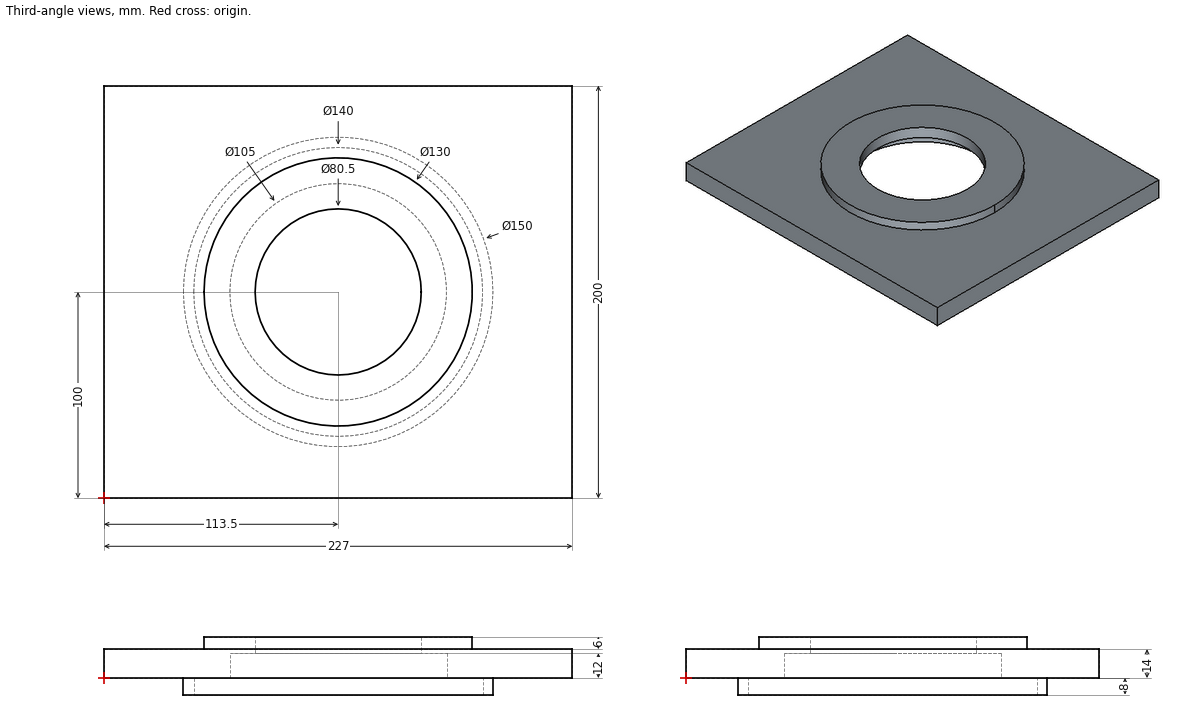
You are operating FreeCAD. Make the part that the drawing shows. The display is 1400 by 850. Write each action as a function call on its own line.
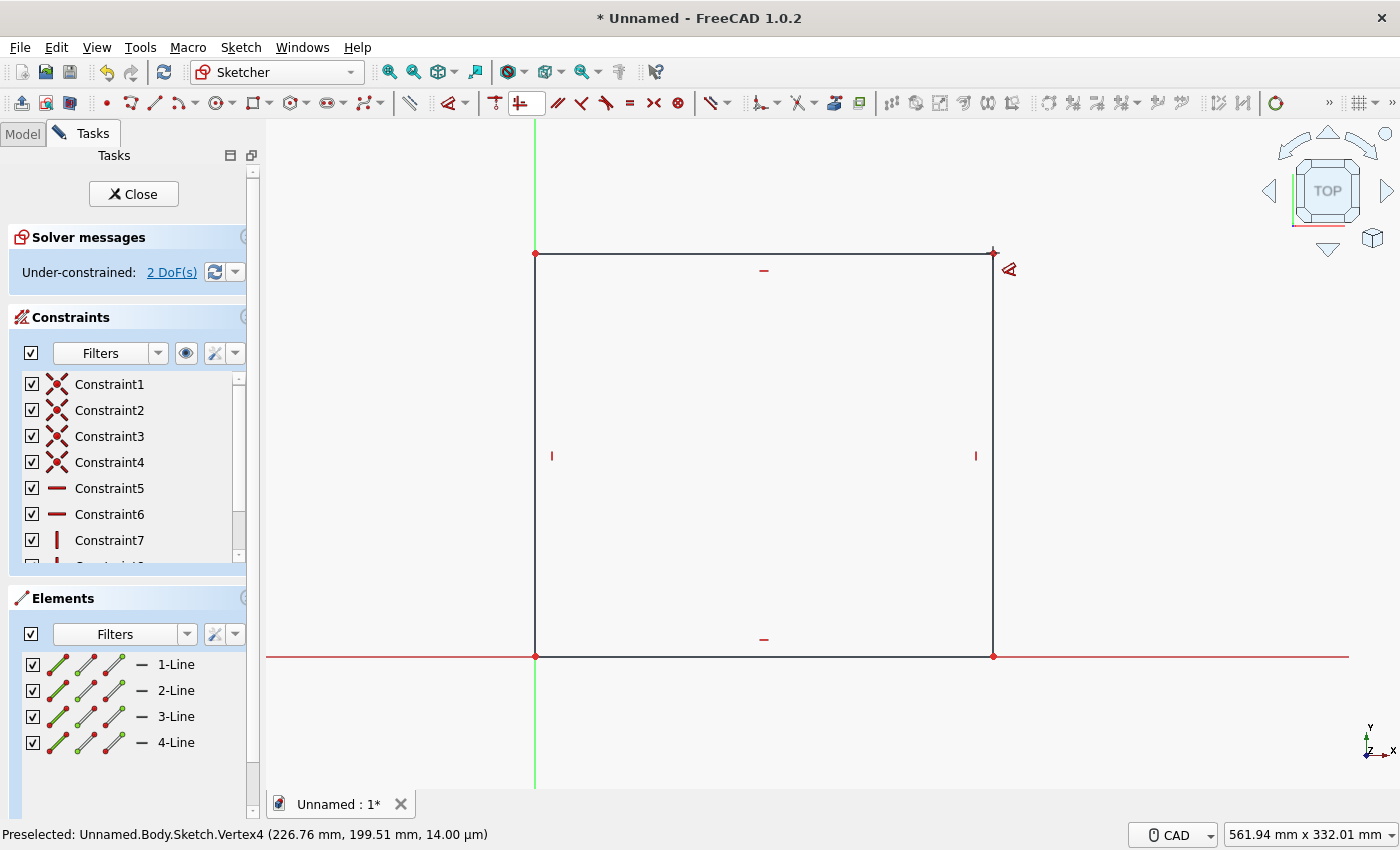
click(673, 657)
click(764, 691)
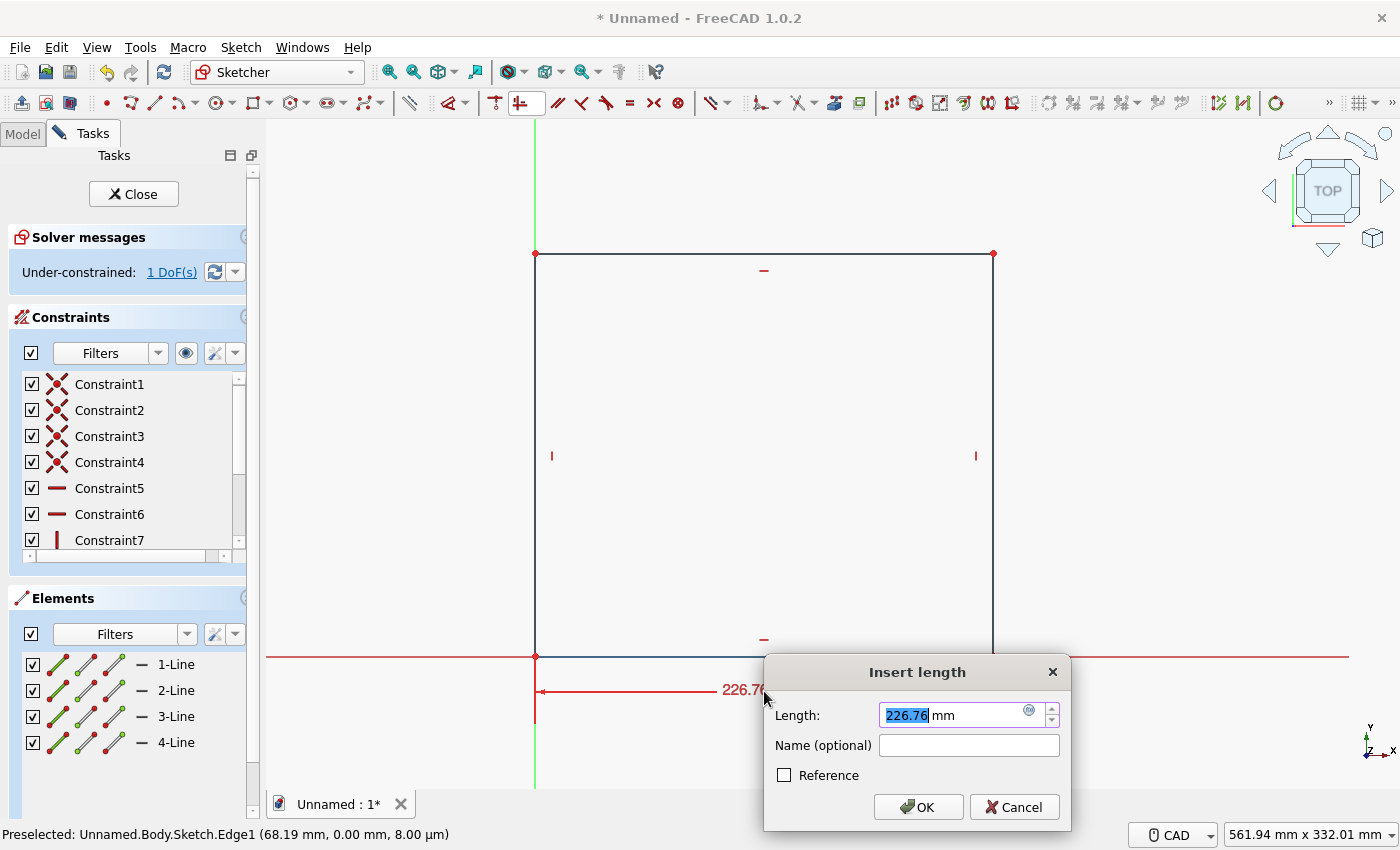
text(227)
key(Return)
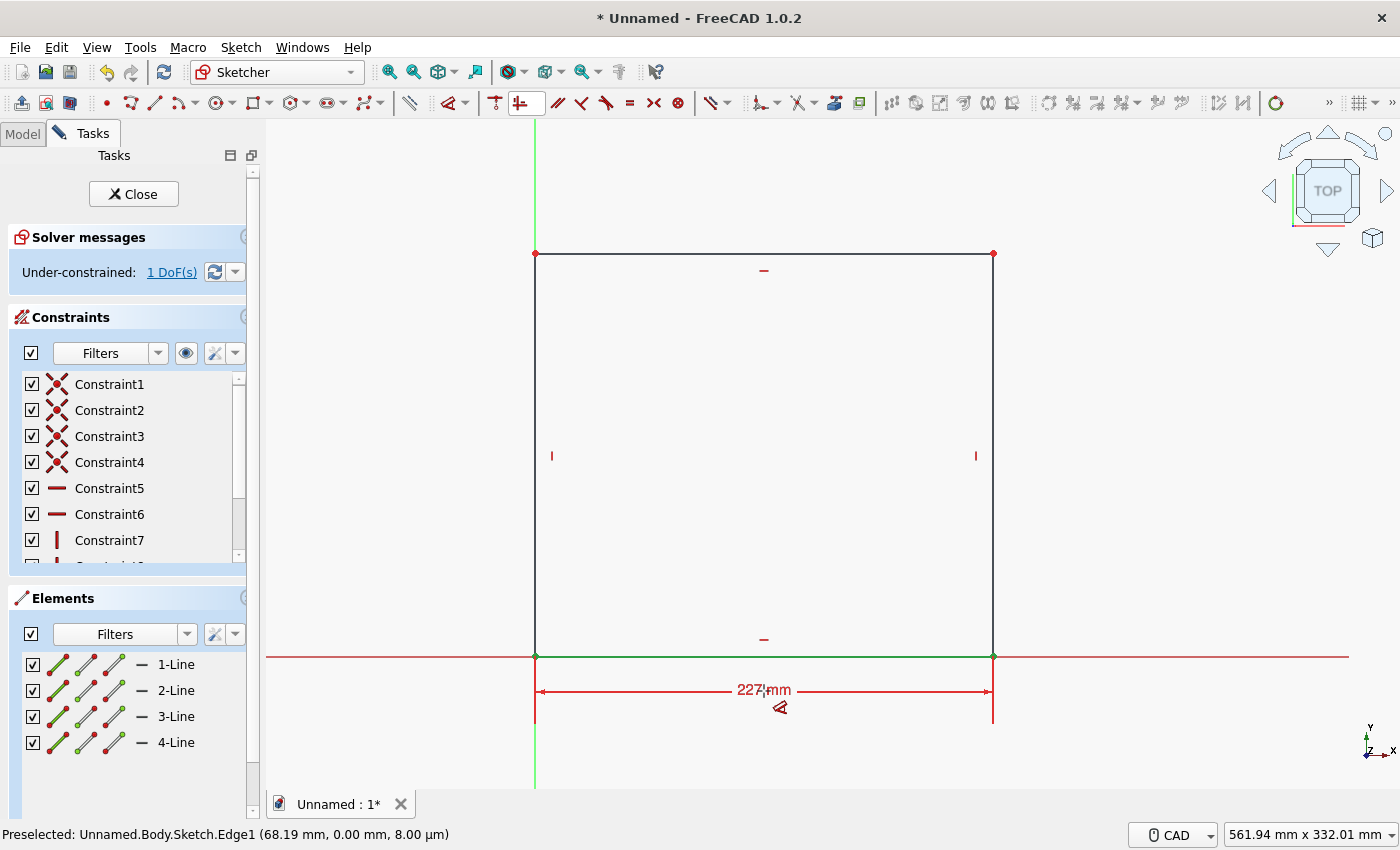
click(993, 536)
click(1027, 455)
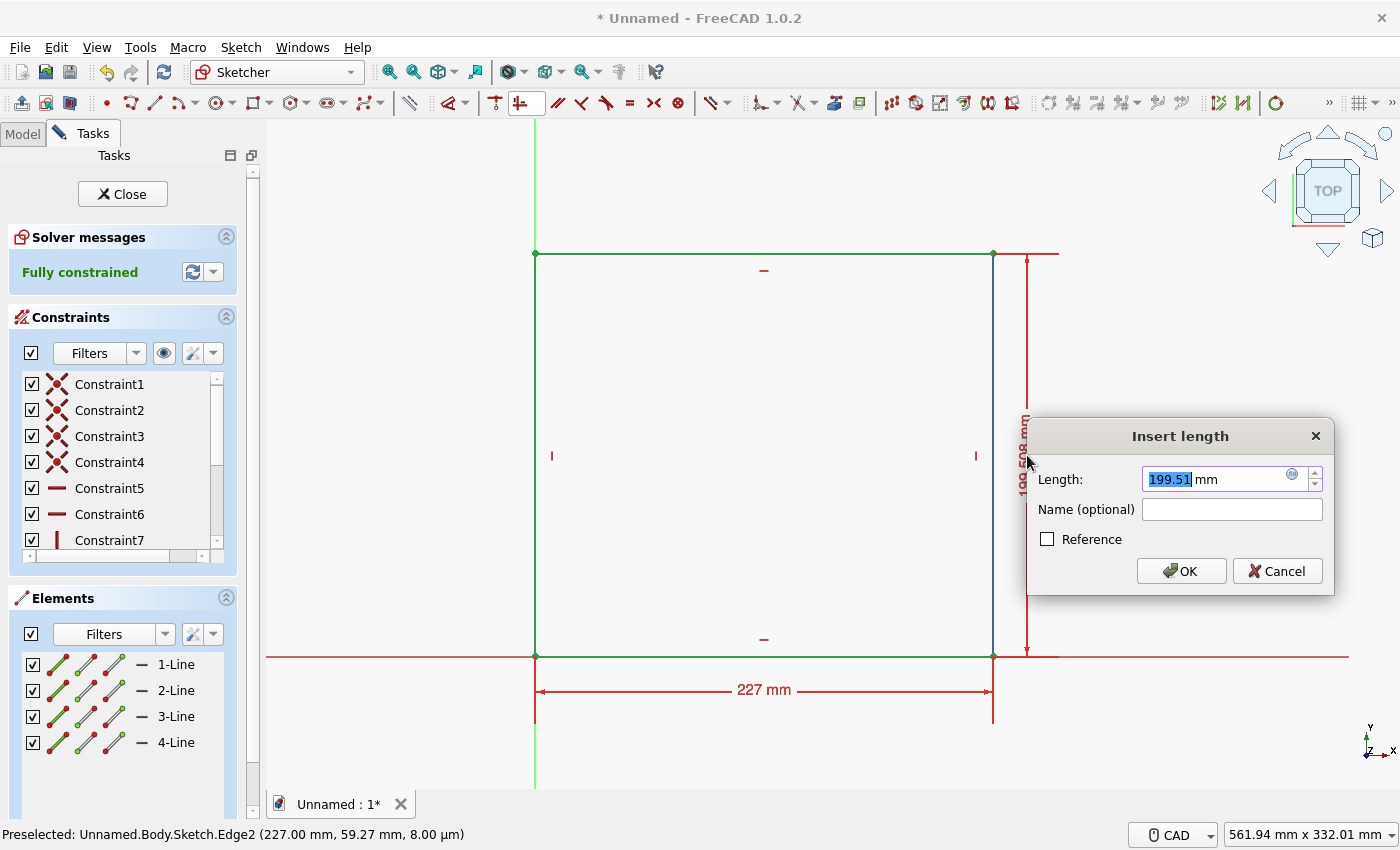
text(200)
key(Return)
key(Escape)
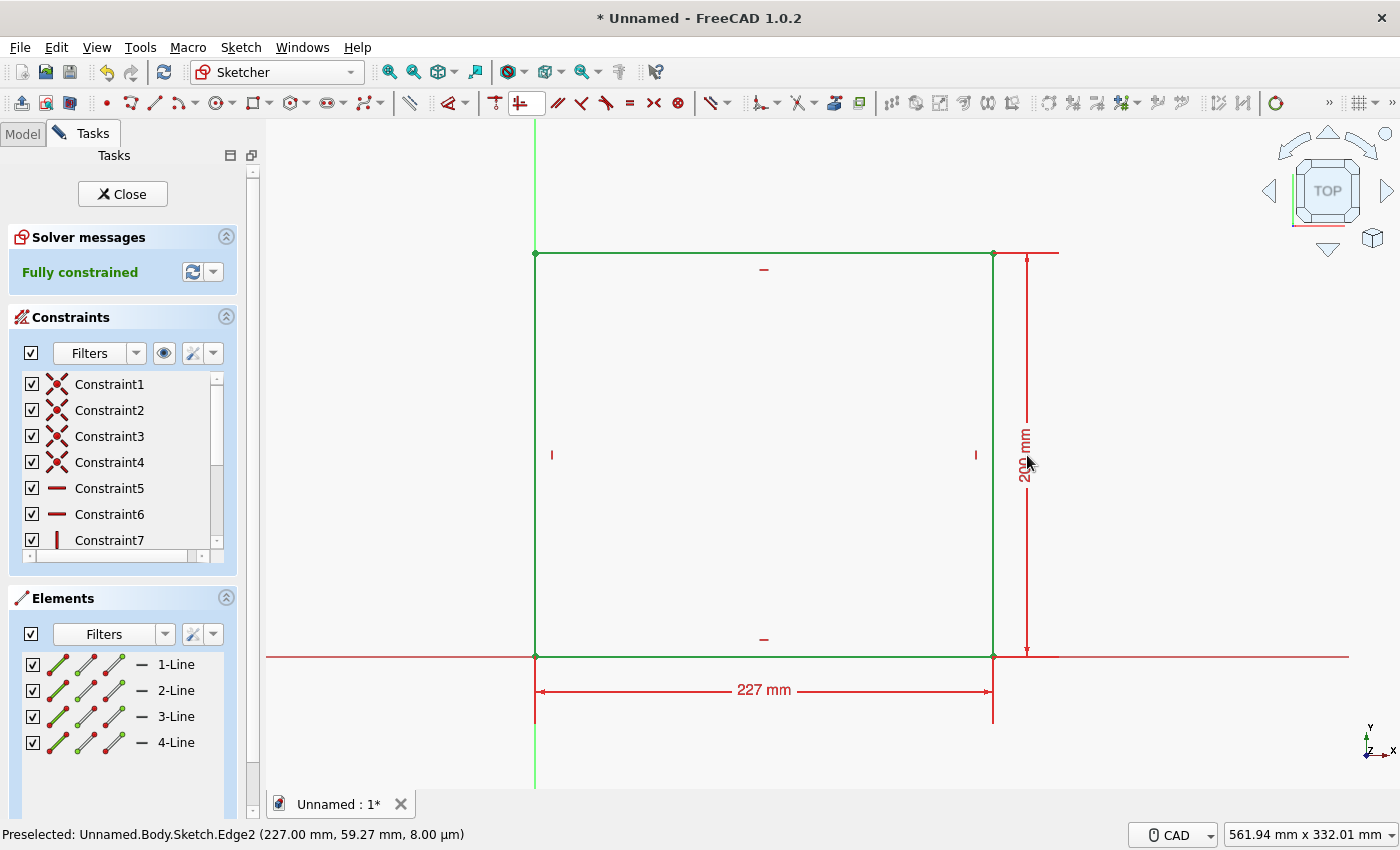
click(123, 194)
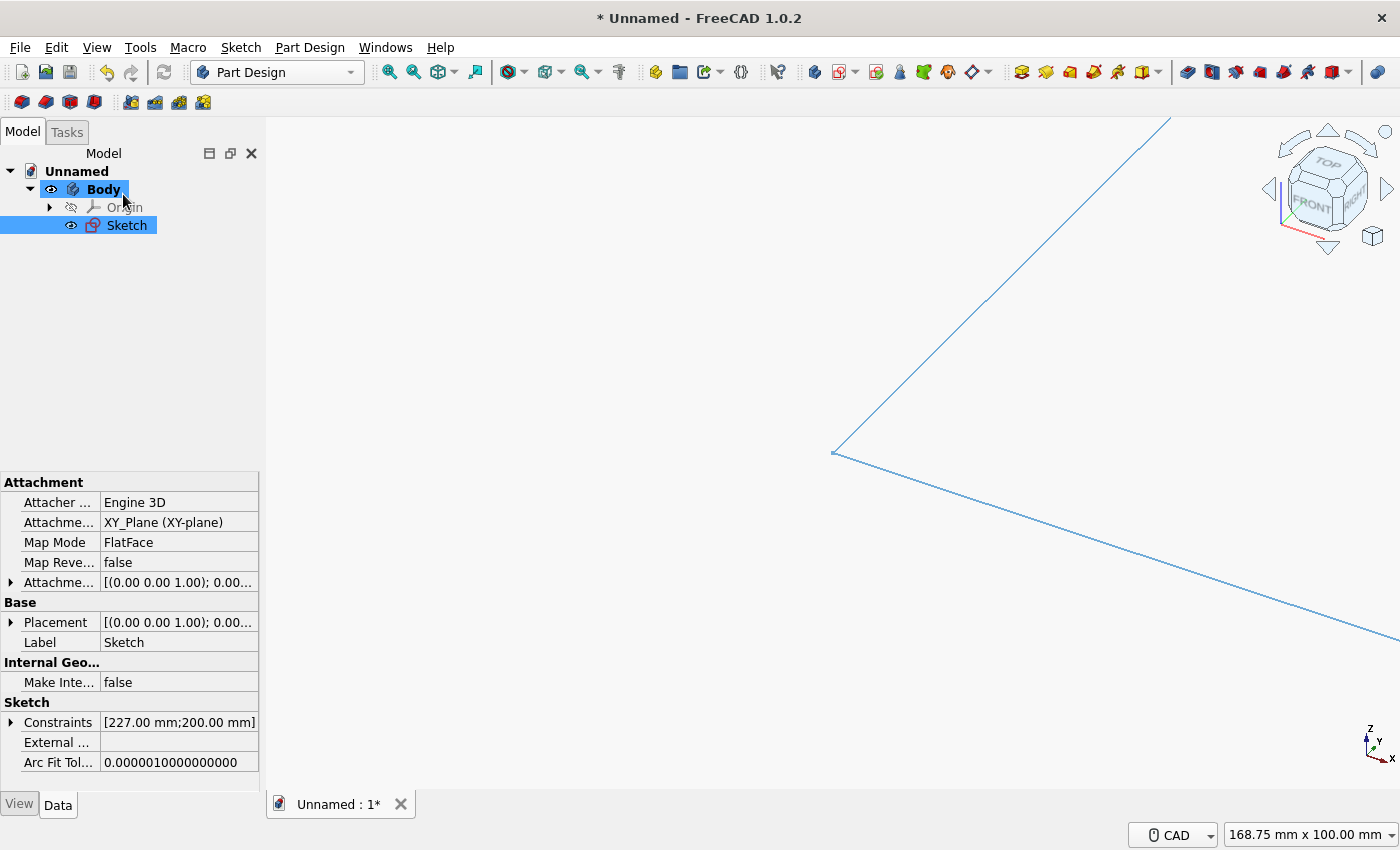
click(1022, 72)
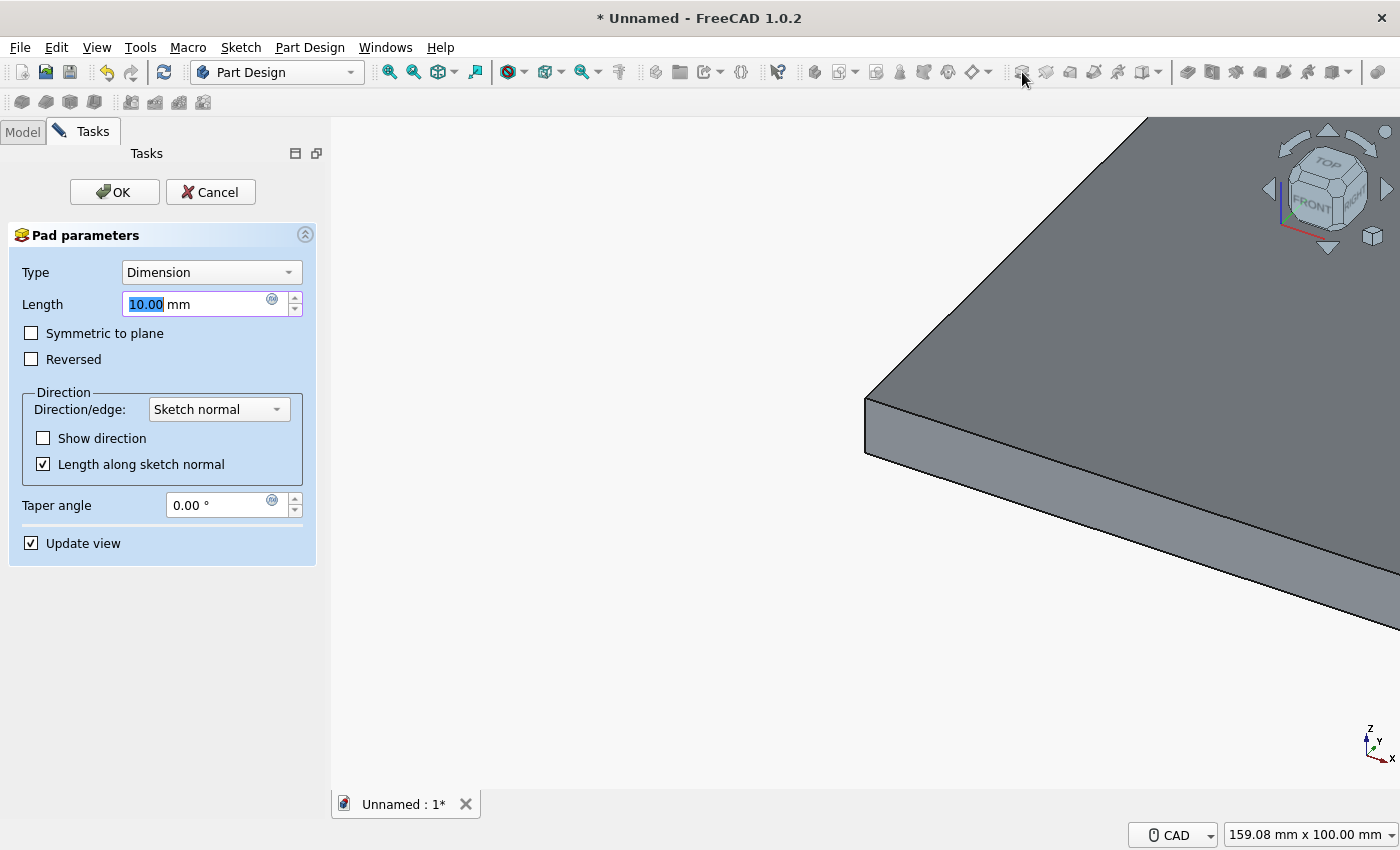
text(14)
key(Tab)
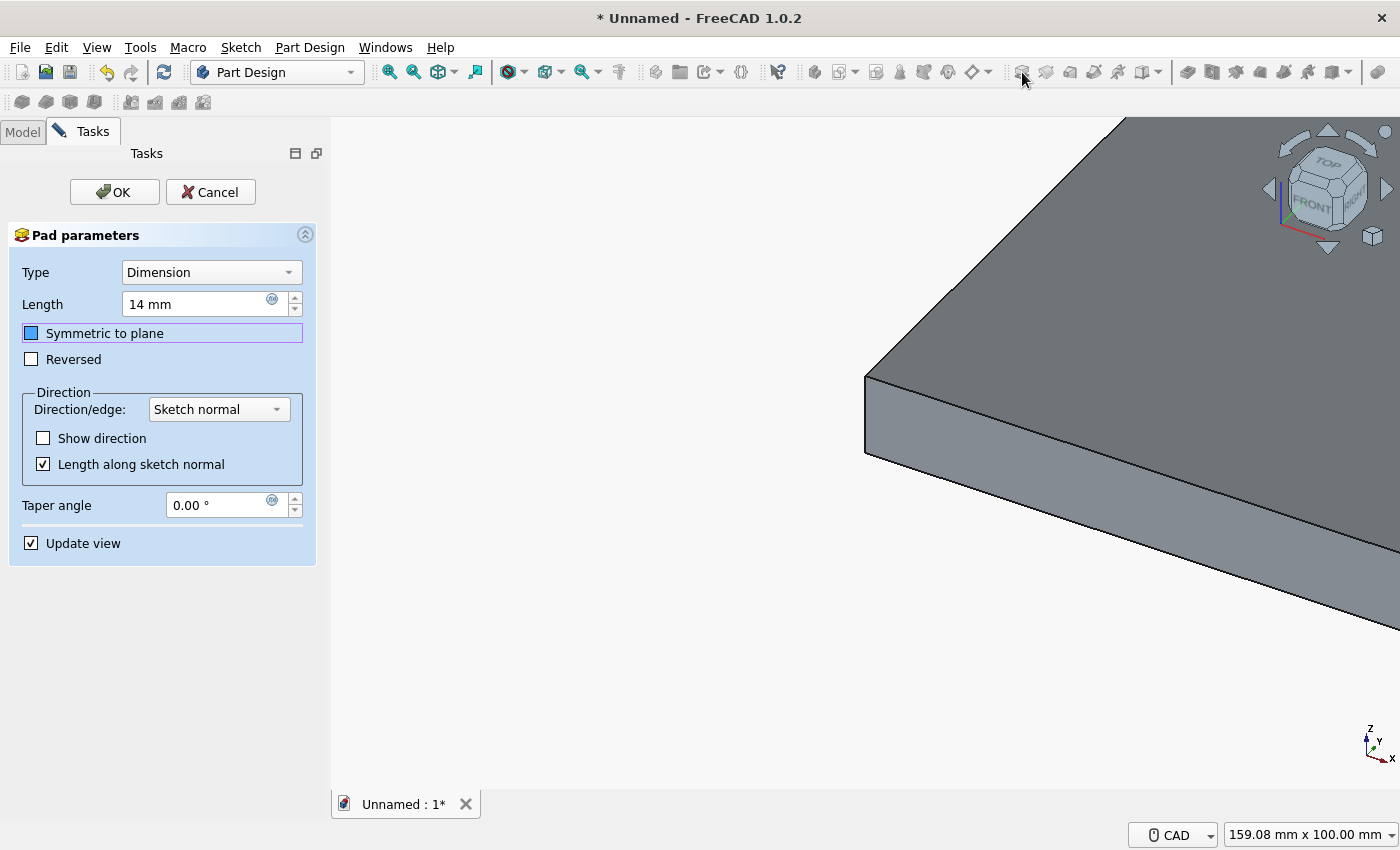
click(115, 192)